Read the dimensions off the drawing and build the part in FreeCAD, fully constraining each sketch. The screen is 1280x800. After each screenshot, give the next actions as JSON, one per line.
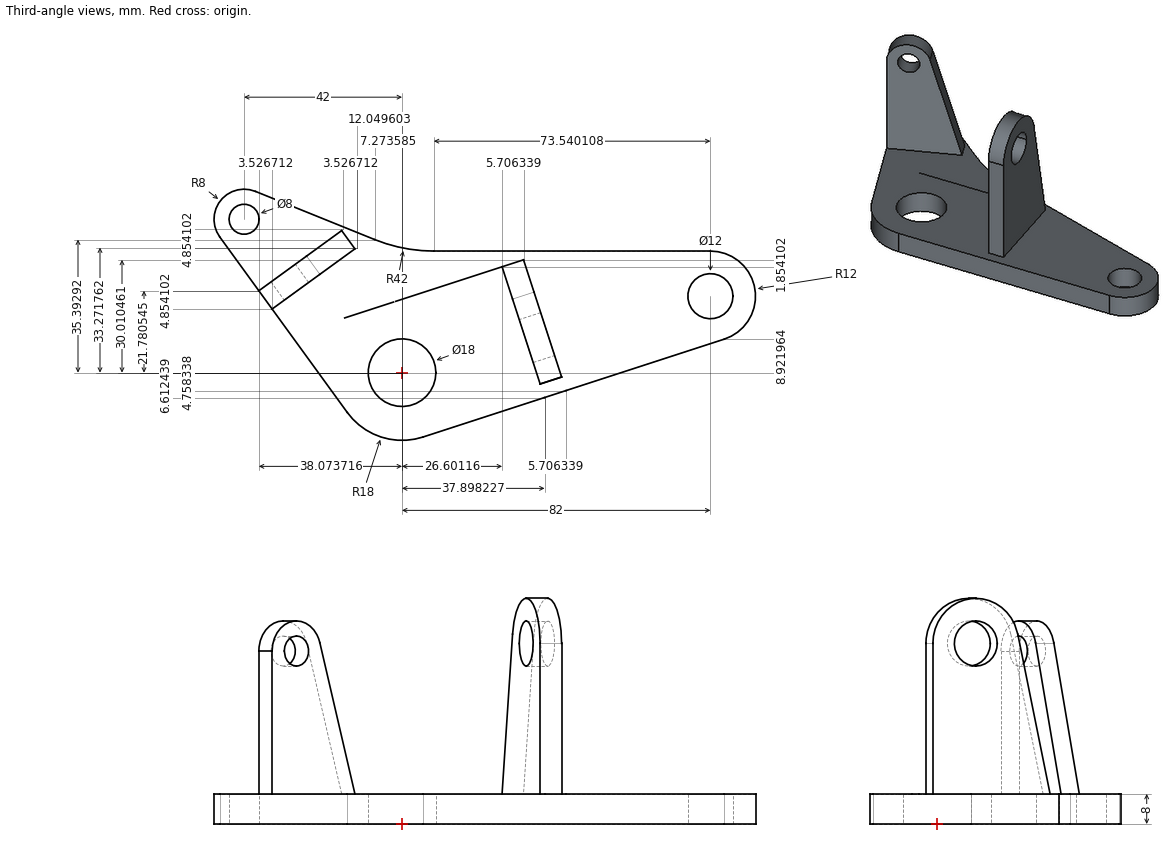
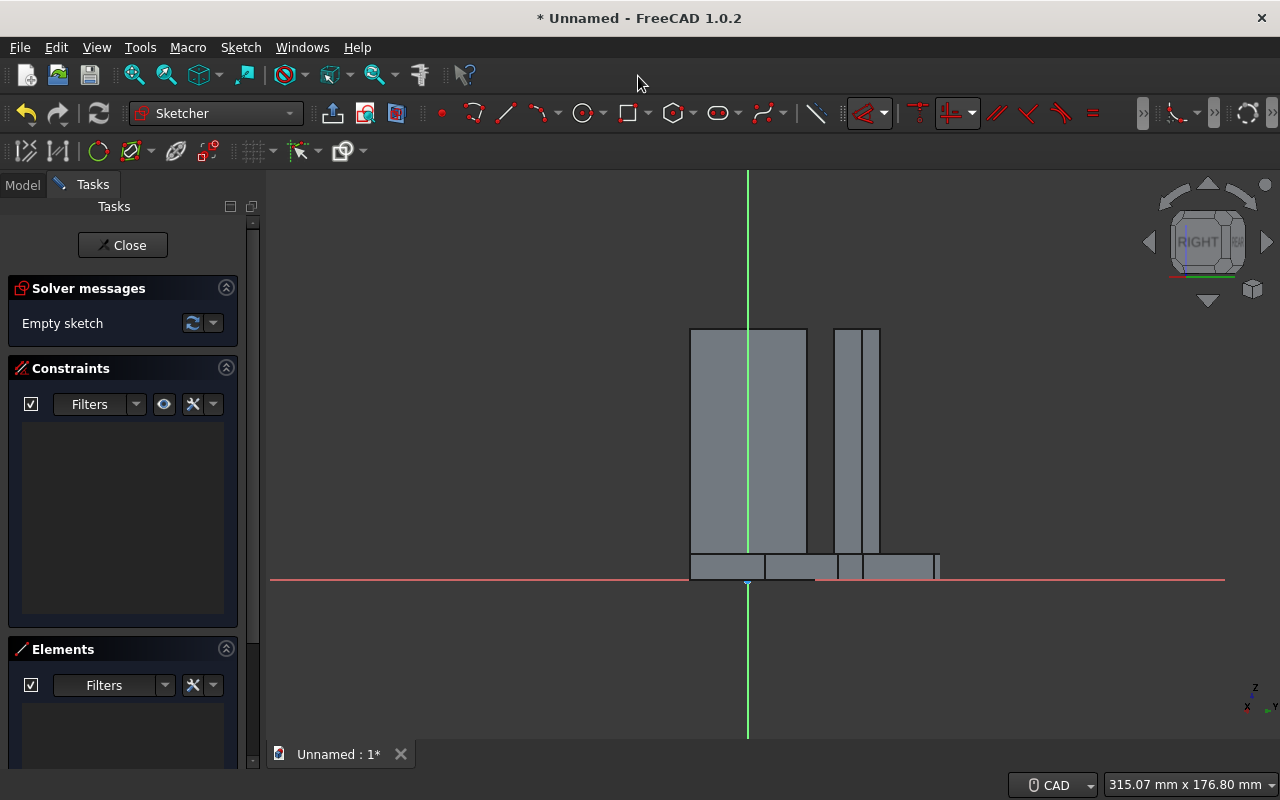
{"action": "scroll", "coordinate": [838, 454], "scroll_direction": "up", "scroll_amount": 2}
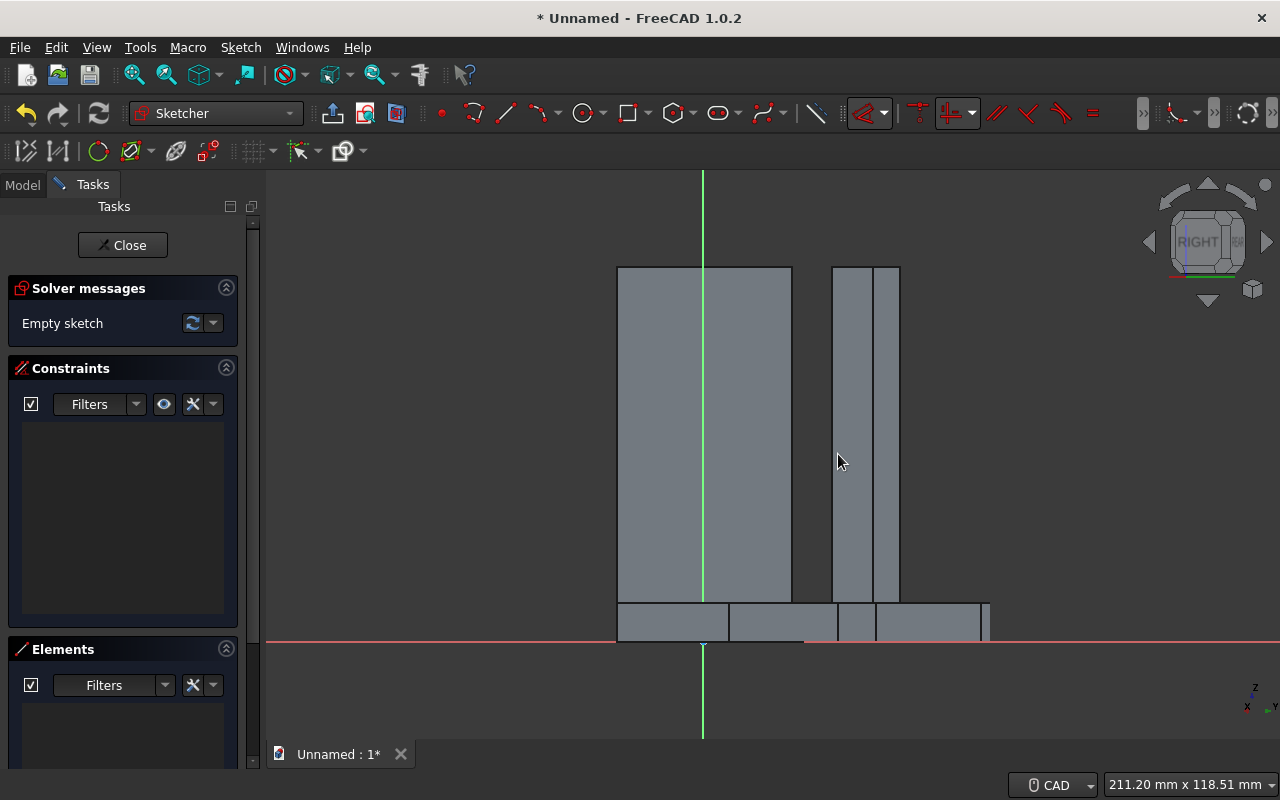
{"action": "key", "text": "g m"}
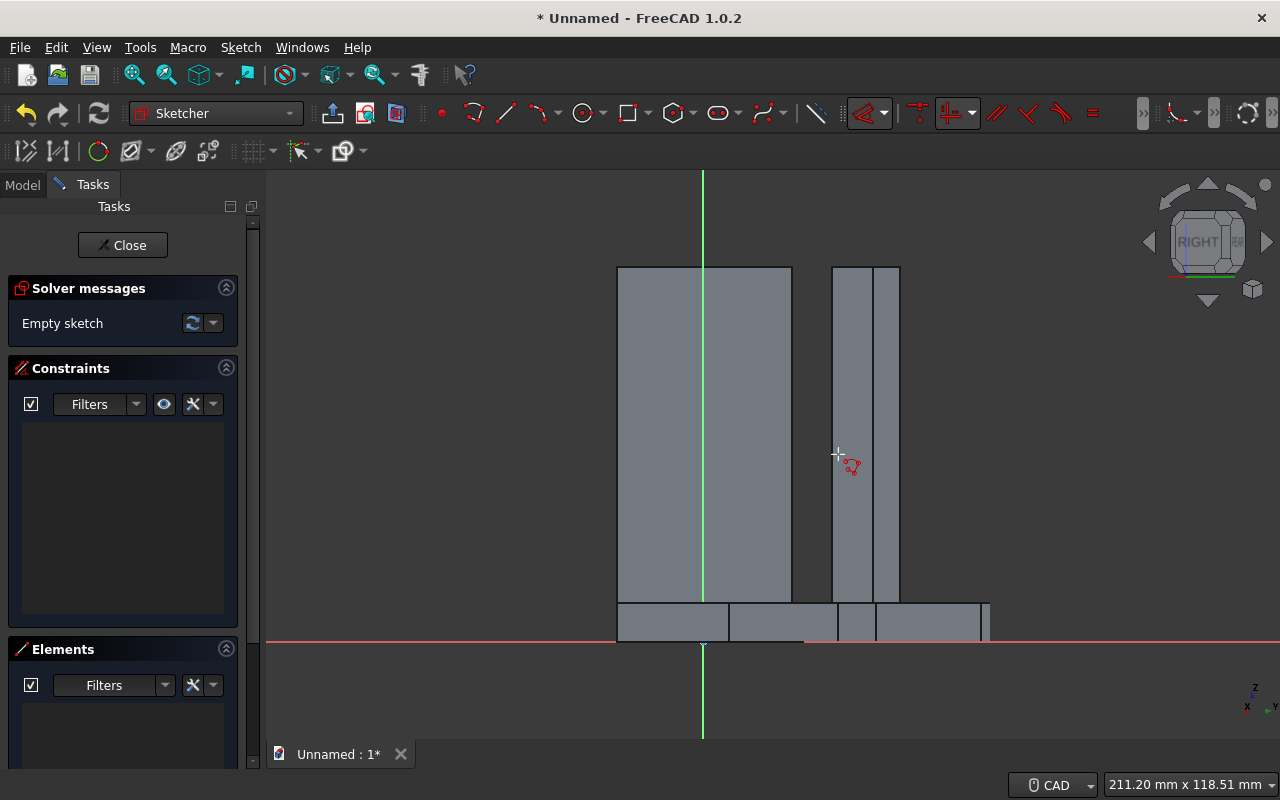
{"action": "left_click", "coordinate": [749, 399]}
{"action": "left_click", "coordinate": [792, 603]}
{"action": "left_click", "coordinate": [792, 267]}
{"action": "left_click", "coordinate": [617, 267]}
{"action": "left_click", "coordinate": [617, 603]}
{"action": "left_click", "coordinate": [635, 603]}
{"action": "left_click", "coordinate": [635, 411]}
{"action": "right_click", "coordinate": [635, 411]}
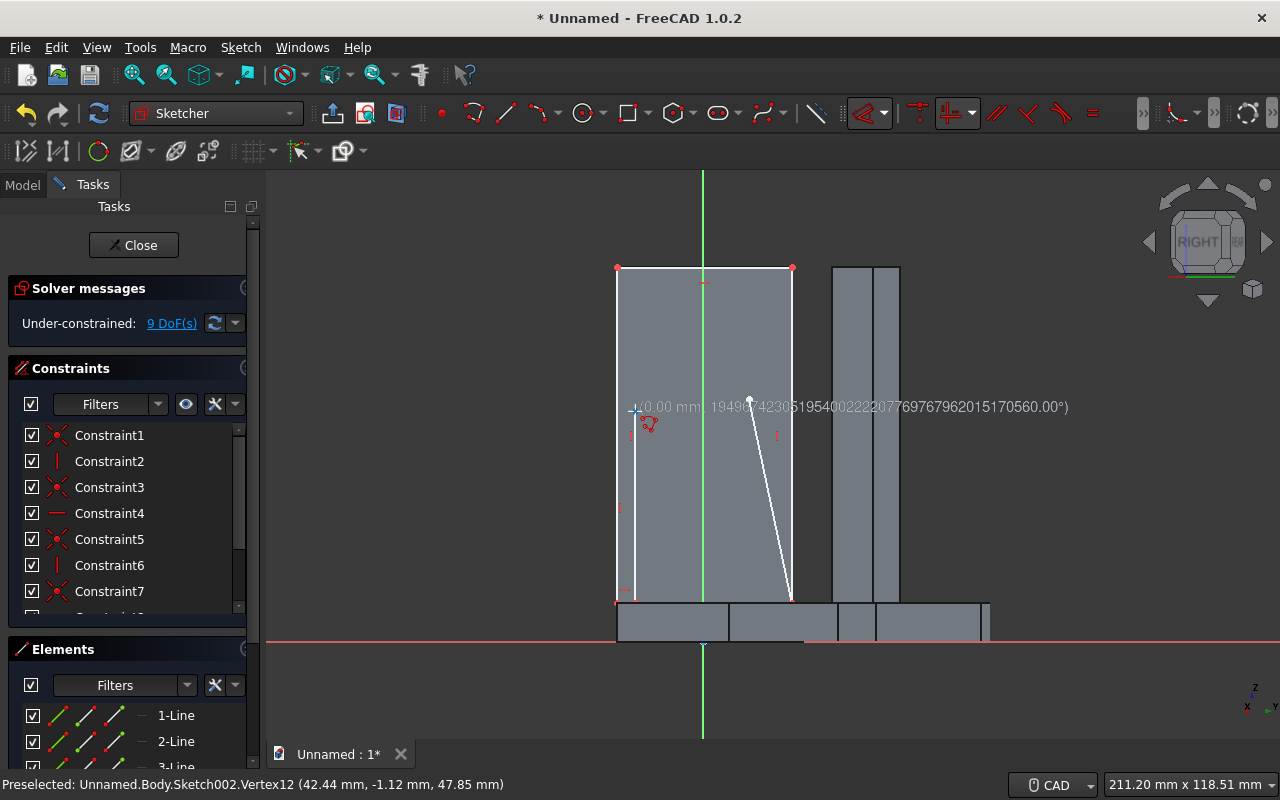
{"action": "key", "text": "g 3 a"}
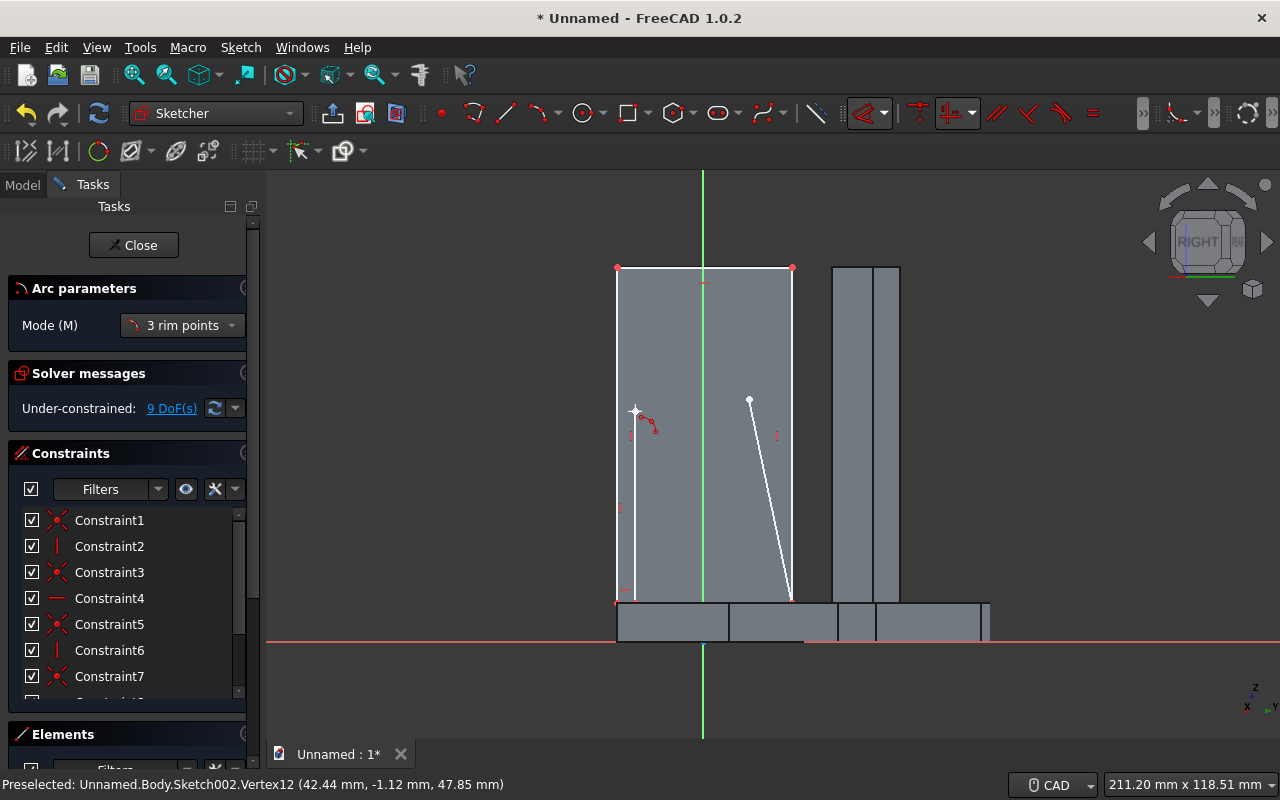
{"action": "left_click", "coordinate": [635, 412]}
{"action": "left_click", "coordinate": [749, 400]}
{"action": "left_click", "coordinate": [686, 354]}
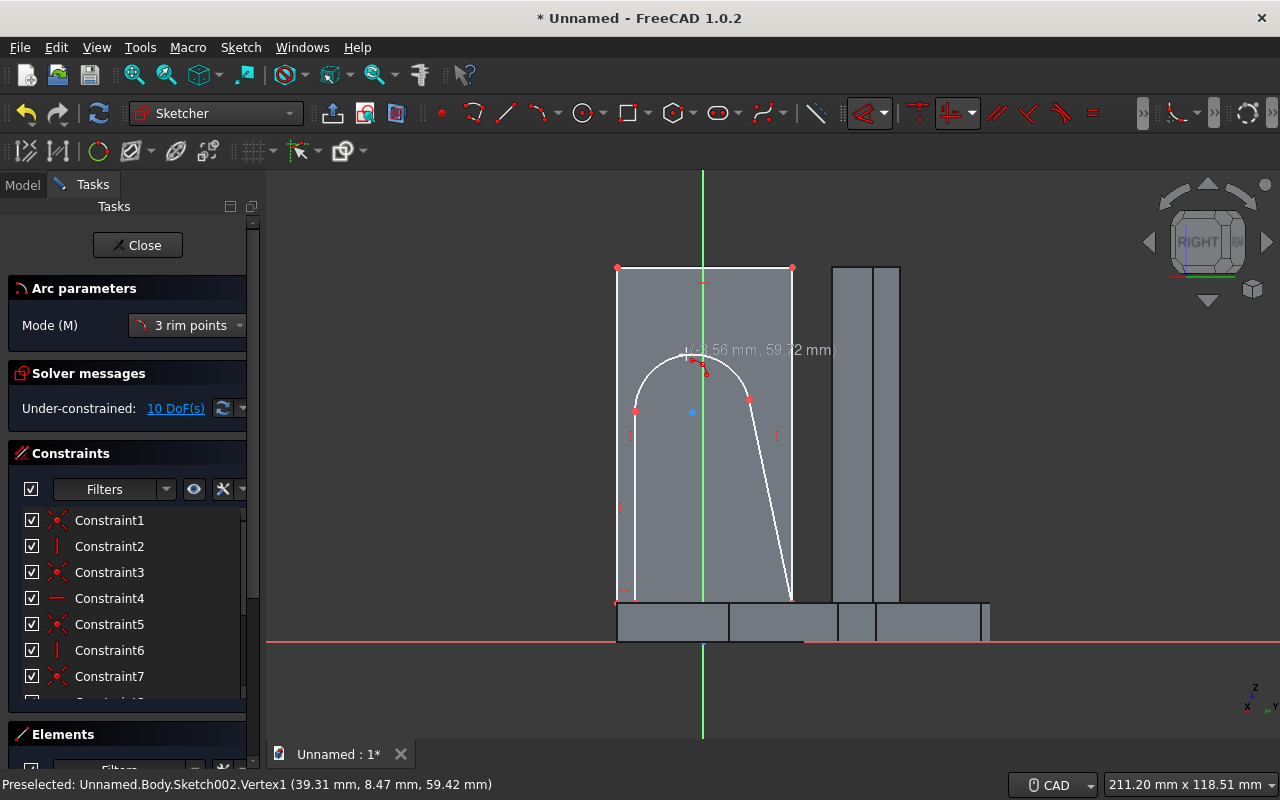
{"action": "key", "text": "g c"}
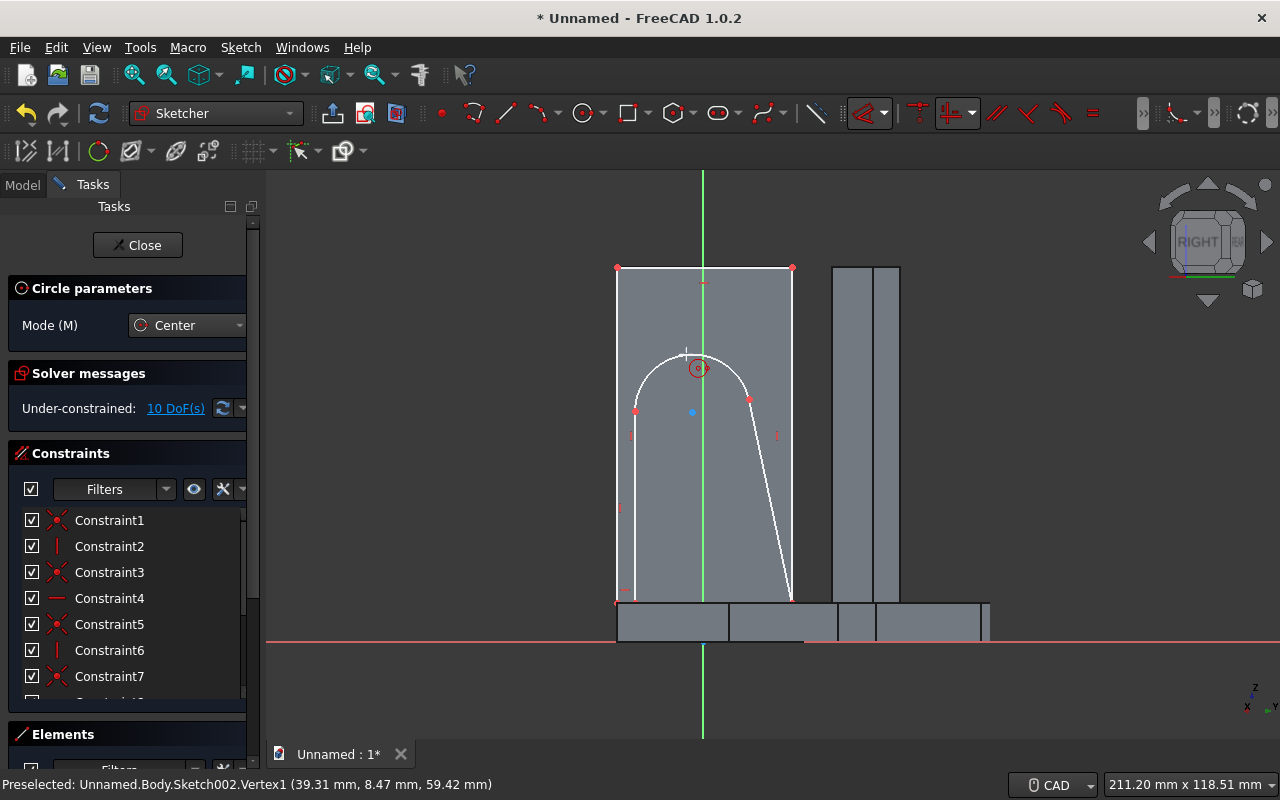
{"action": "scroll", "coordinate": [692, 411], "scroll_direction": "up", "scroll_amount": 3}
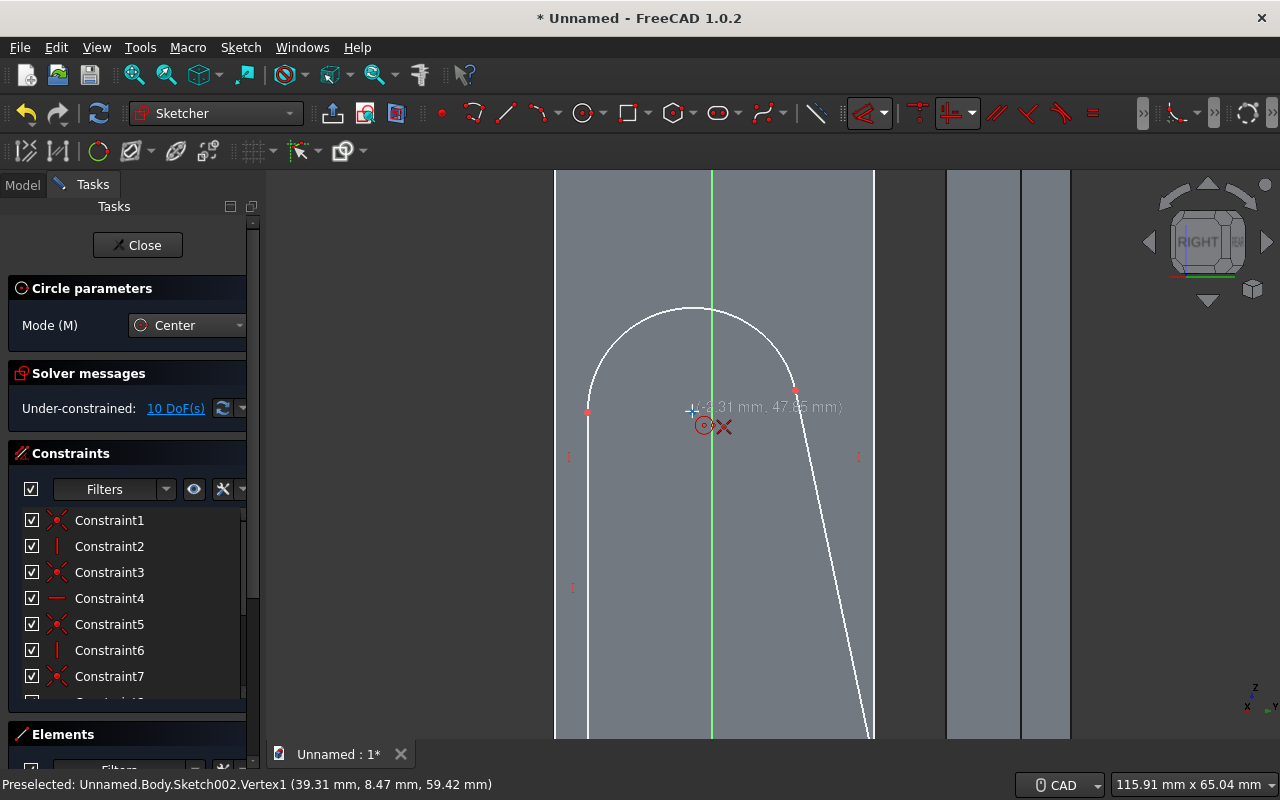
{"action": "left_click", "coordinate": [693, 411]}
{"action": "left_click", "coordinate": [730, 374]}
{"action": "key", "text": "Escape"}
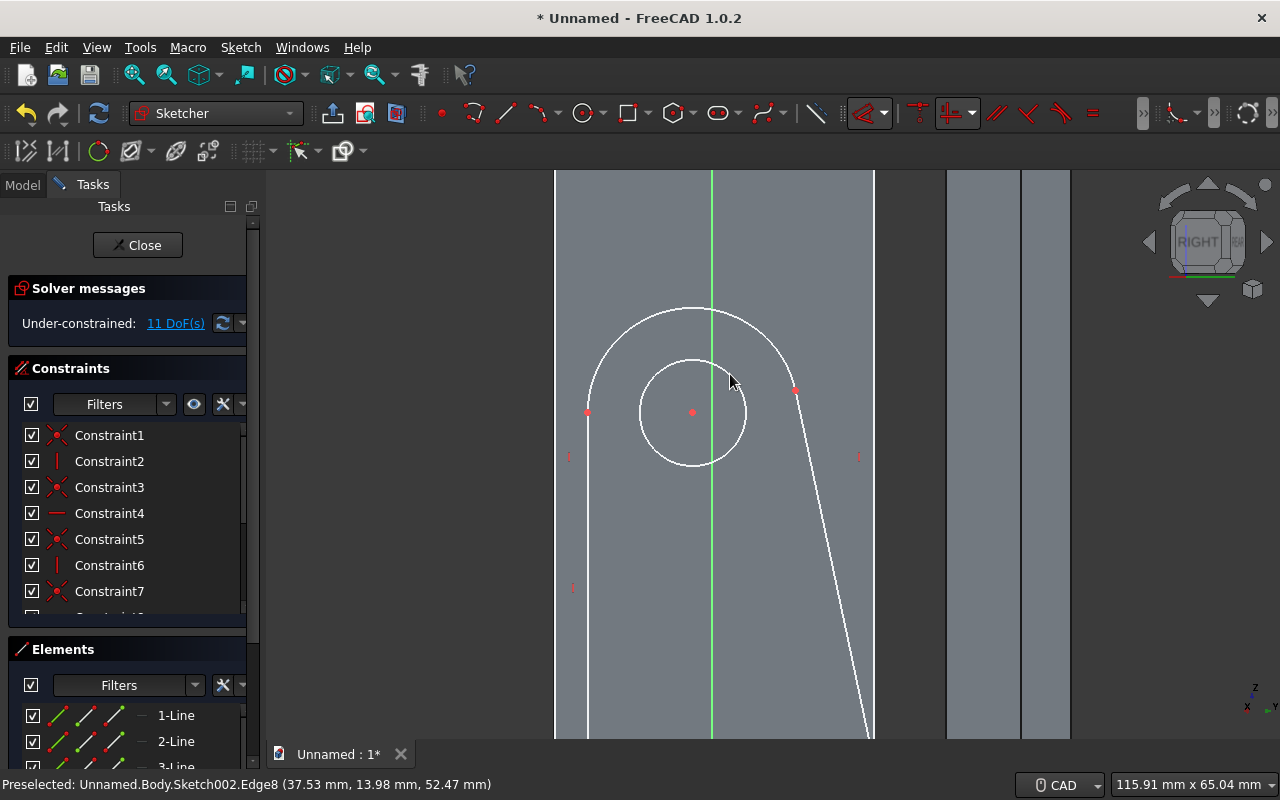
{"action": "left_click", "coordinate": [819, 502]}